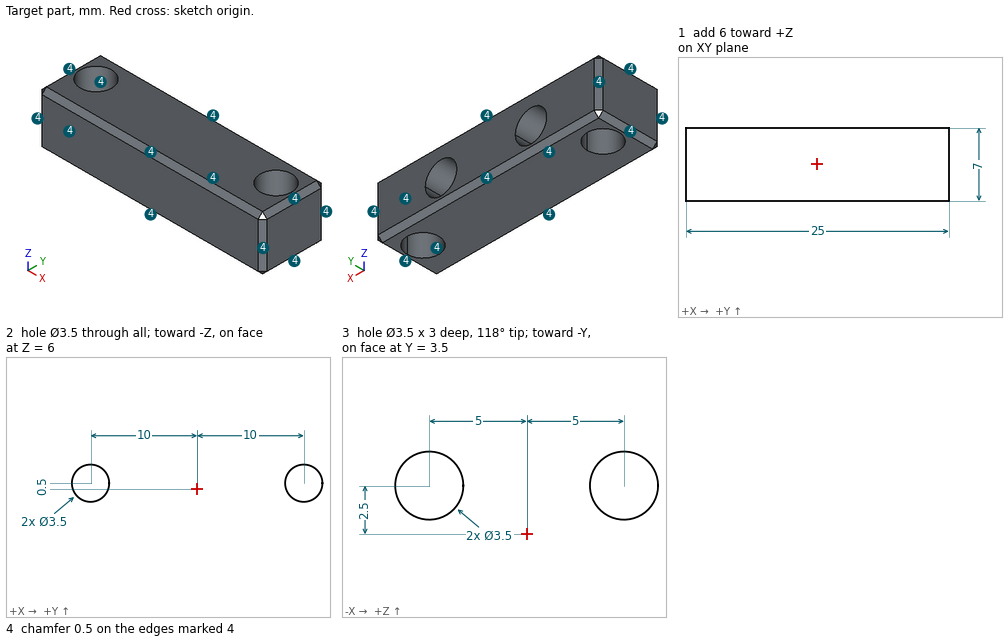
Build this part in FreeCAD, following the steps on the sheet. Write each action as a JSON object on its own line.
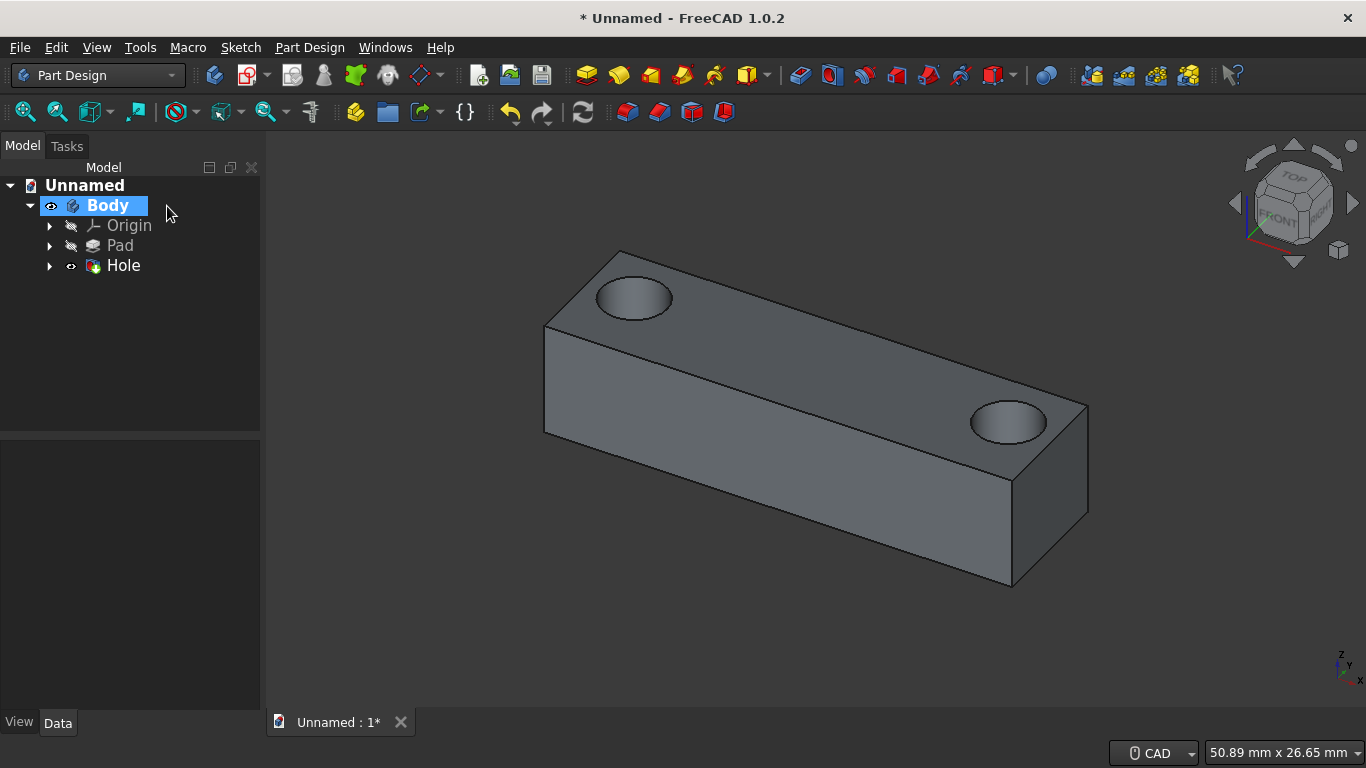
{"action": "key", "text": "4"}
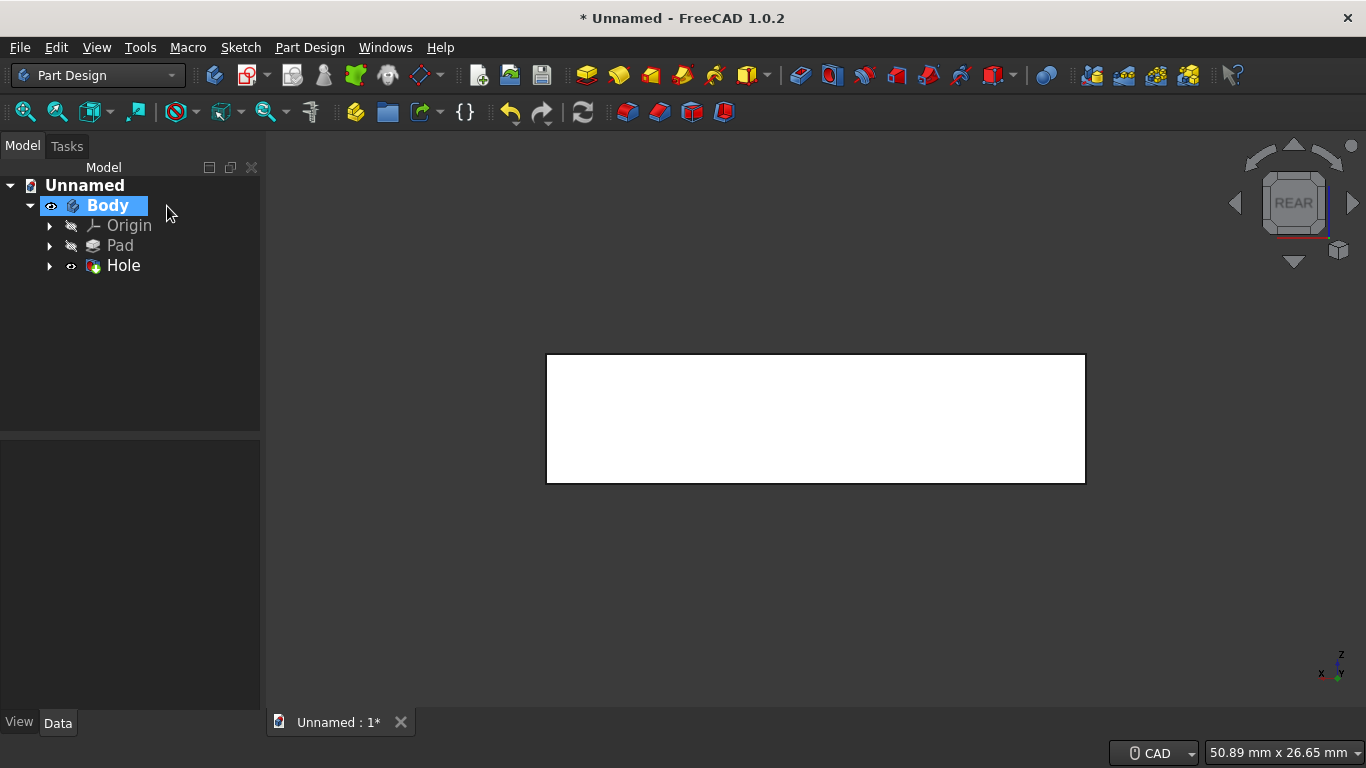
{"action": "left_click", "coordinate": [662, 418]}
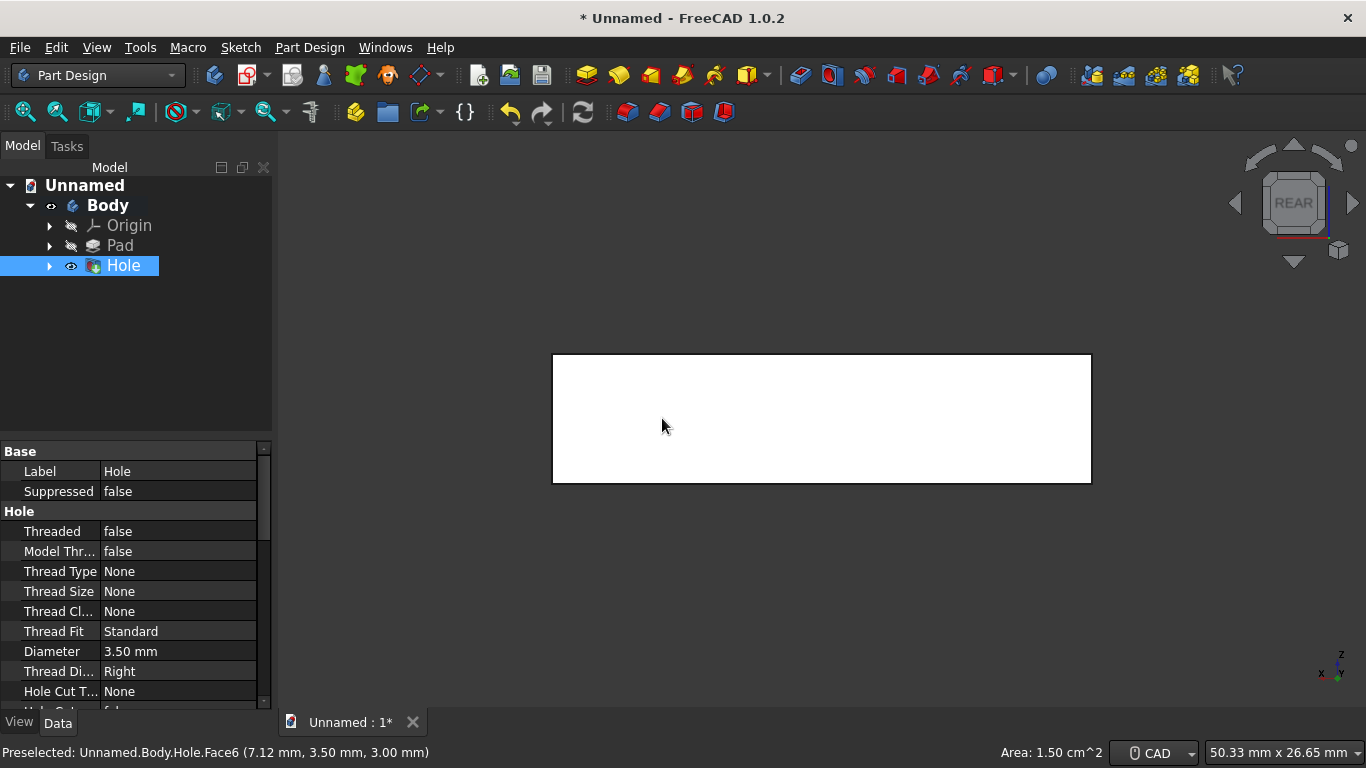
{"action": "left_click", "coordinate": [248, 76]}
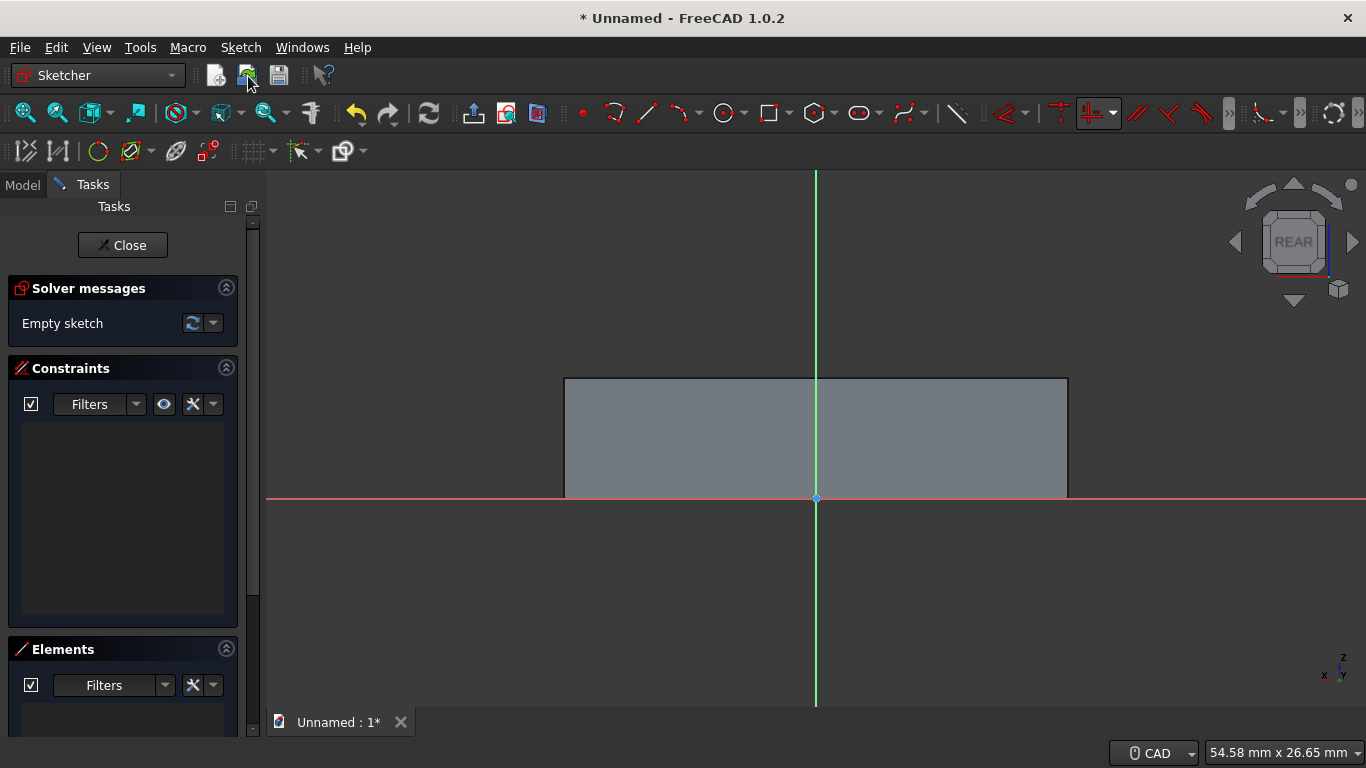
{"action": "scroll", "coordinate": [872, 471], "scroll_direction": "up", "scroll_amount": 4}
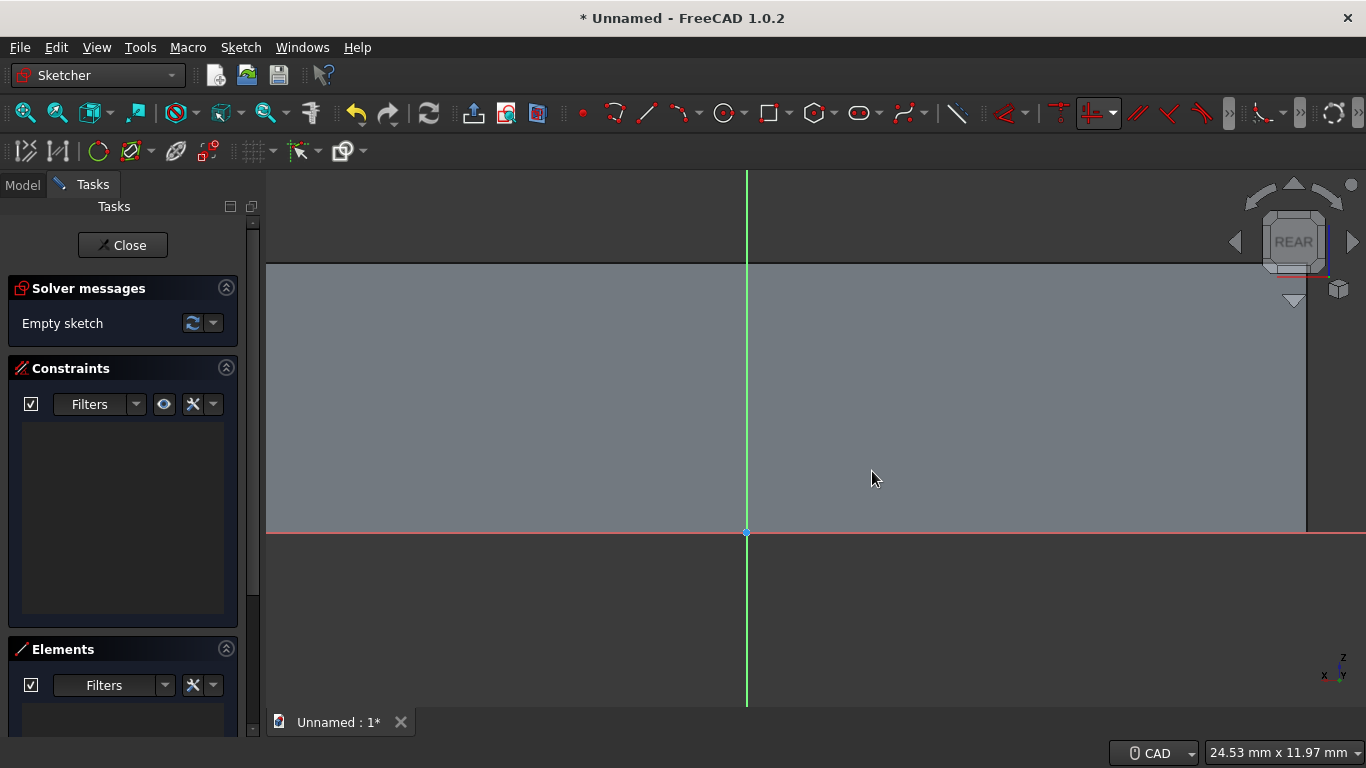
{"action": "left_click", "coordinate": [724, 114]}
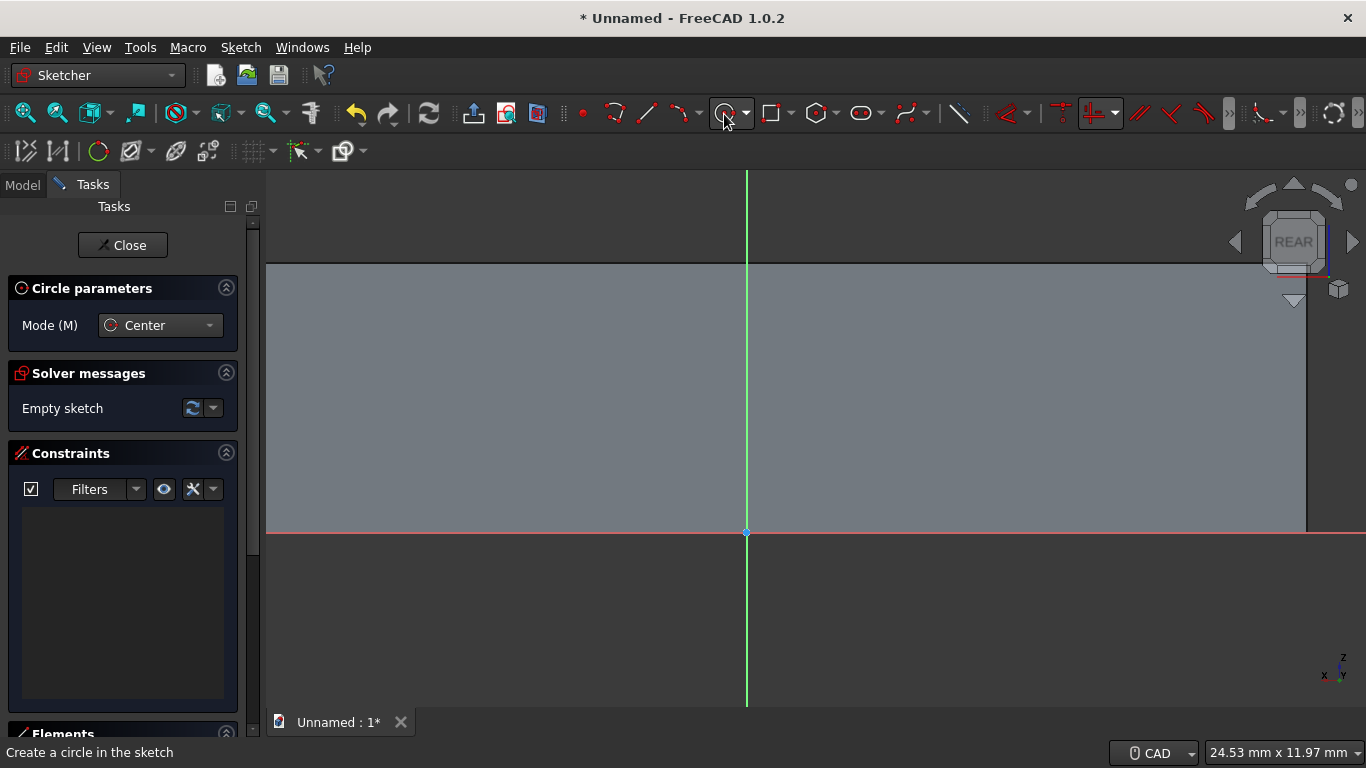
{"action": "left_click", "coordinate": [522, 420]}
{"action": "mouse_move", "coordinate": [578, 365]}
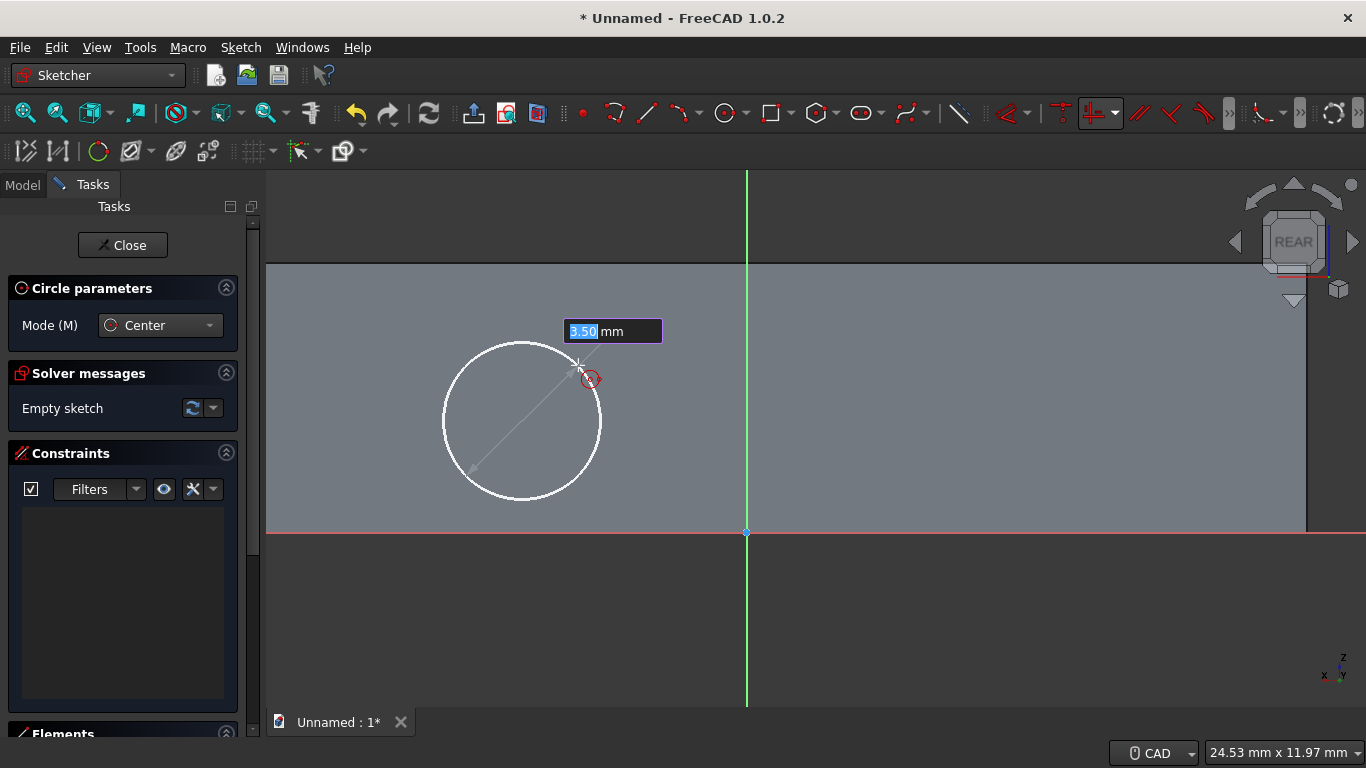
{"action": "type", "text": "3.5"}
{"action": "key", "text": "Return"}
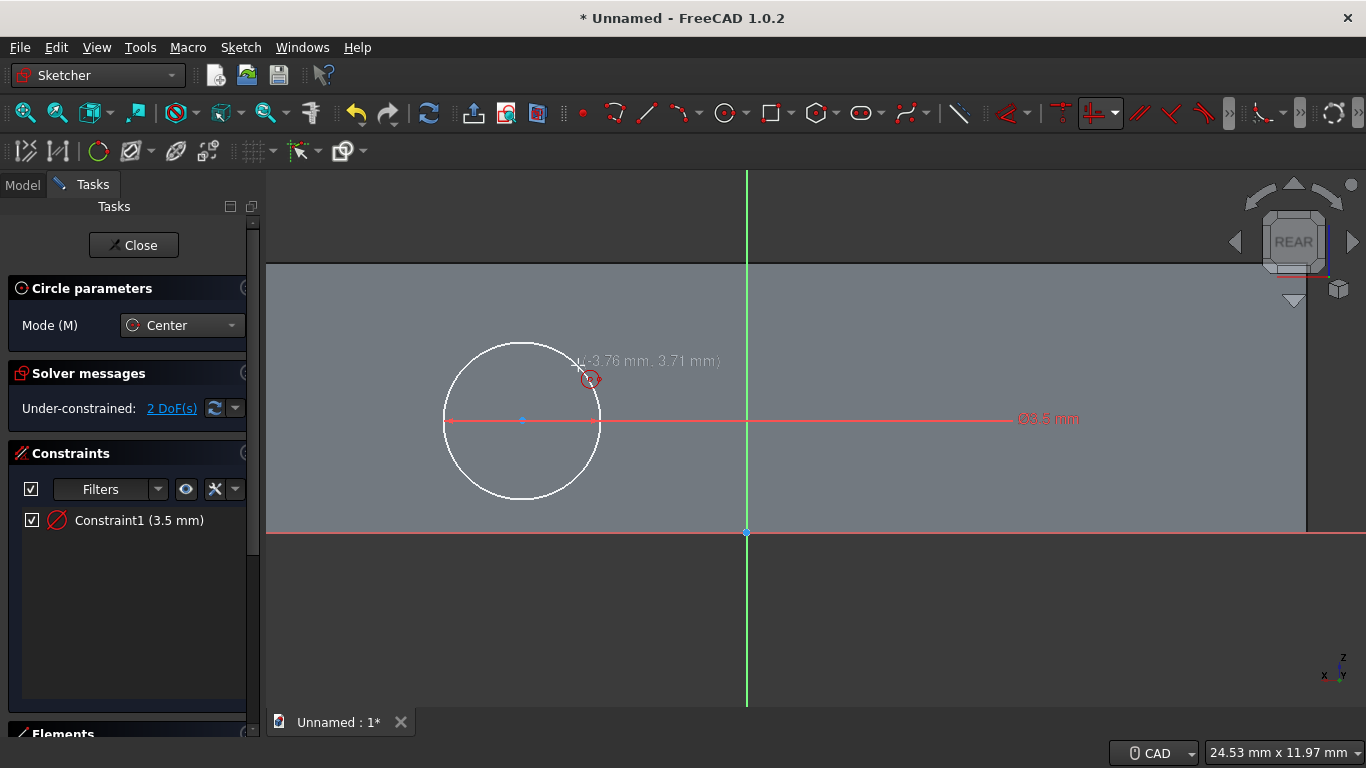
{"action": "left_click", "coordinate": [971, 420]}
{"action": "mouse_move", "coordinate": [1026, 365]}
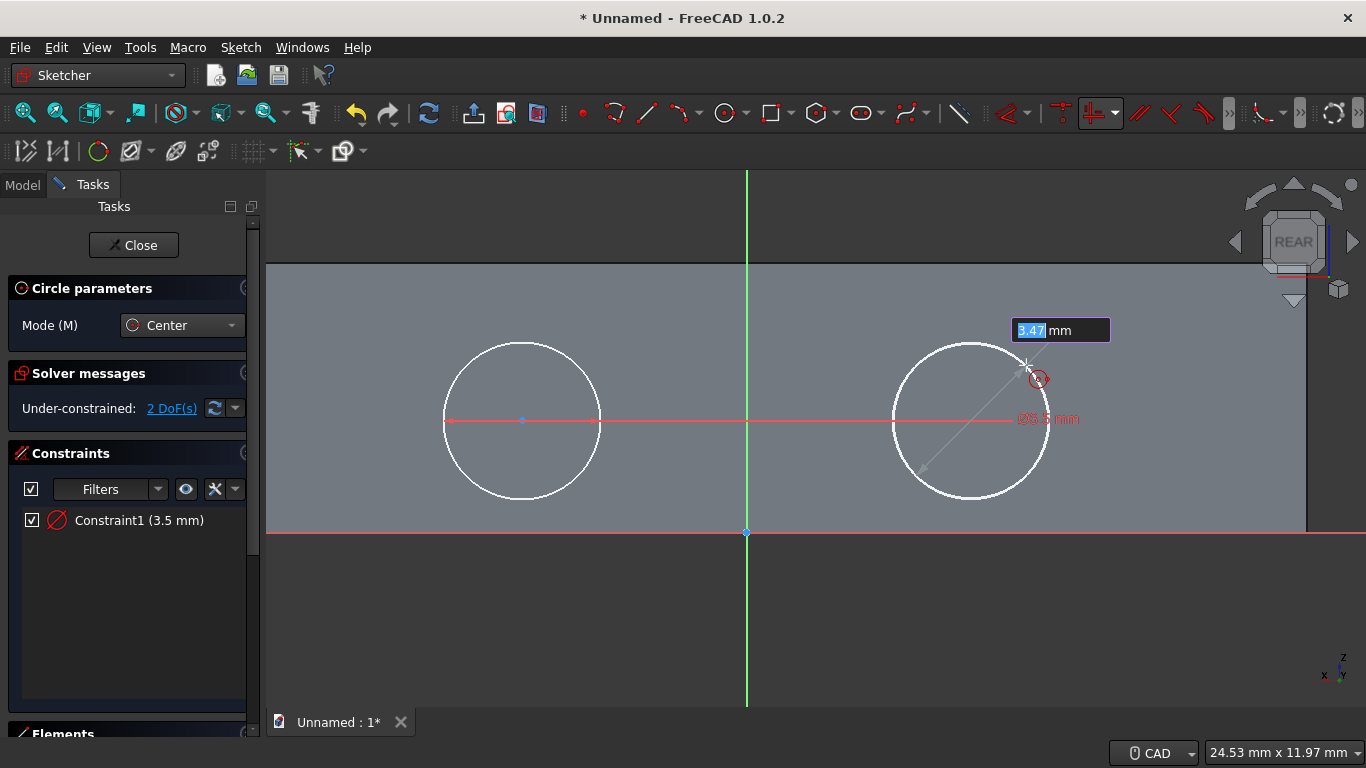
{"action": "type", "text": "3.5"}
{"action": "key", "text": "Return"}
{"action": "key", "text": "Escape"}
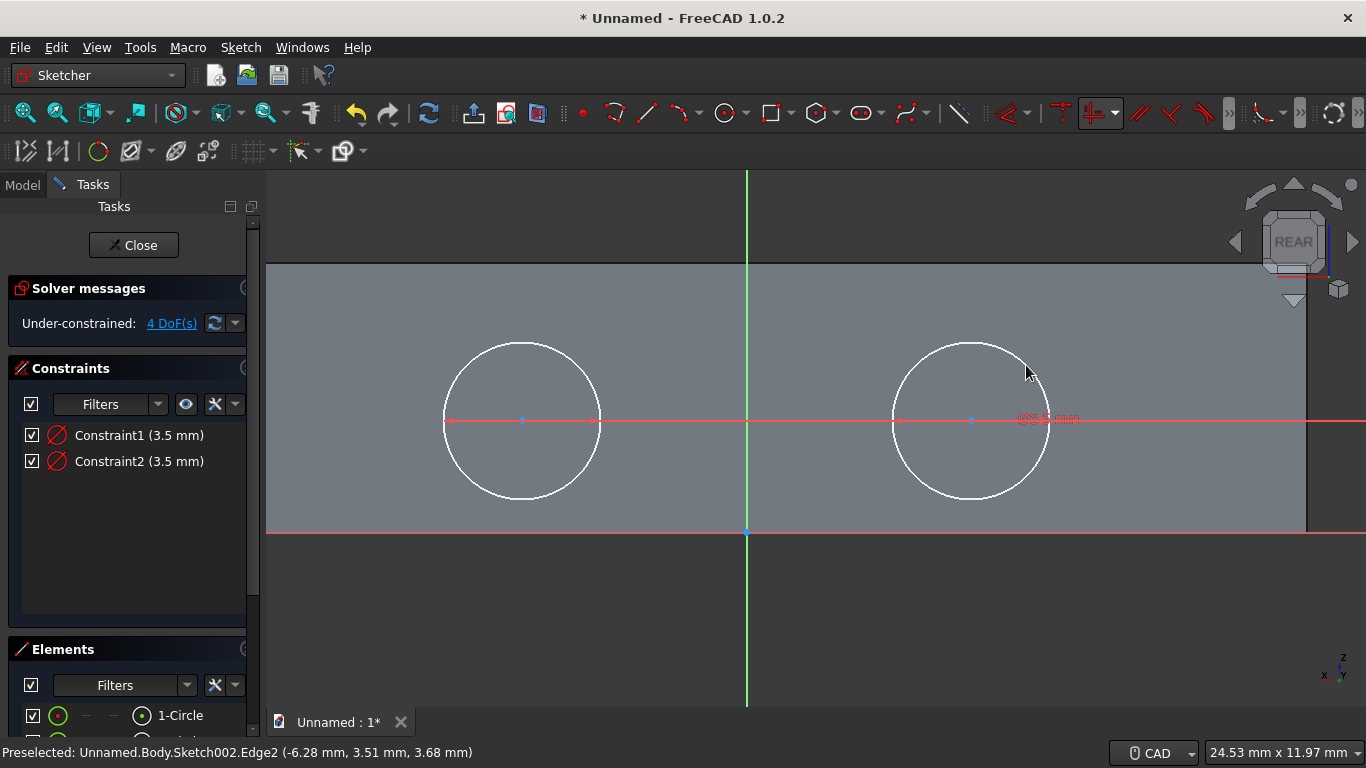
{"action": "left_click", "coordinate": [522, 421]}